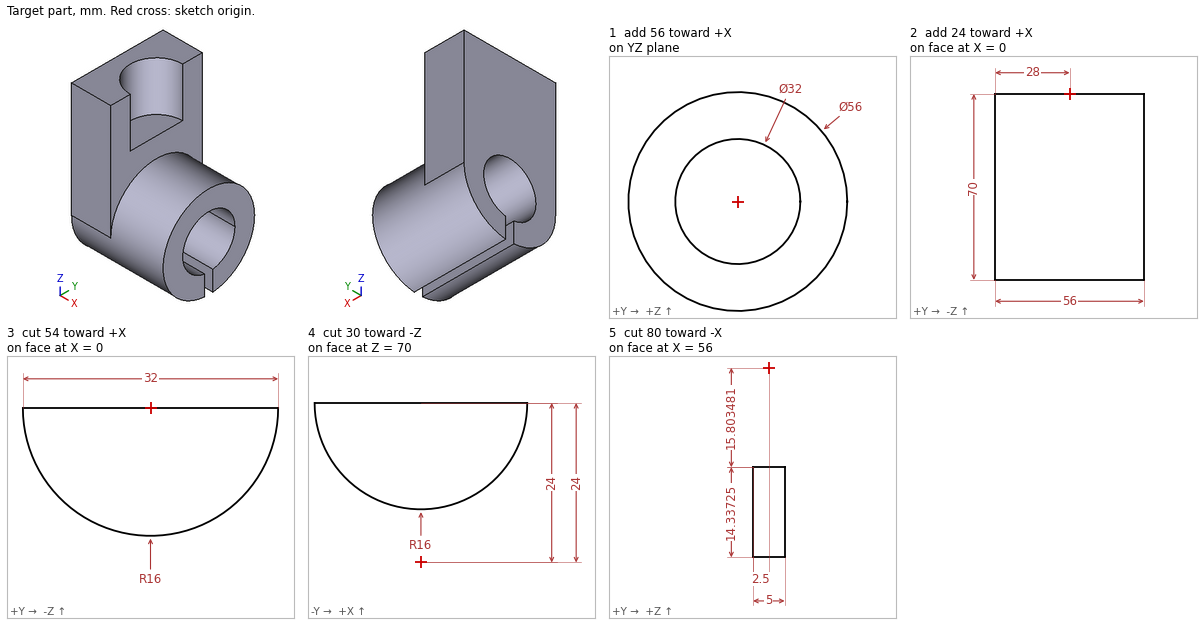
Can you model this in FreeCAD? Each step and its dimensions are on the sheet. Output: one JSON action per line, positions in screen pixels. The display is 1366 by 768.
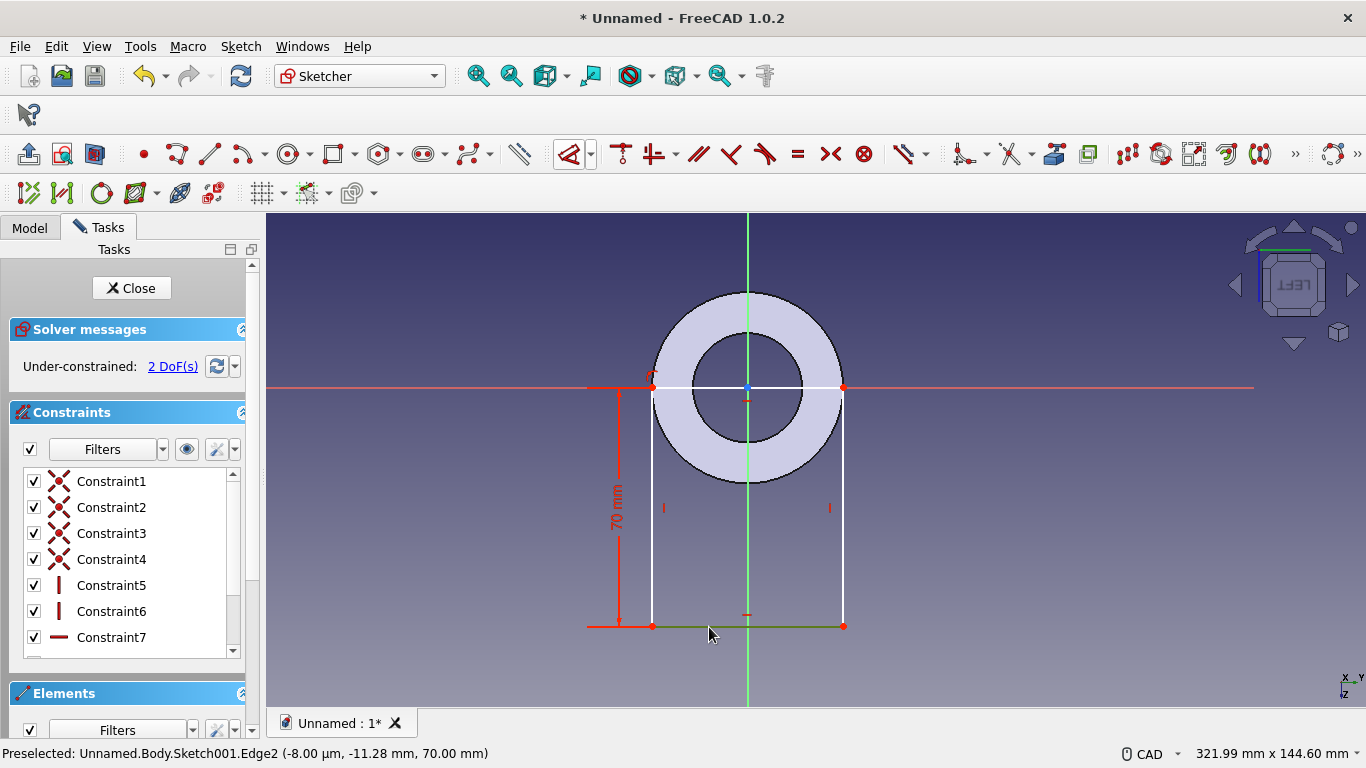
{"action": "left_click", "coordinate": [590, 154]}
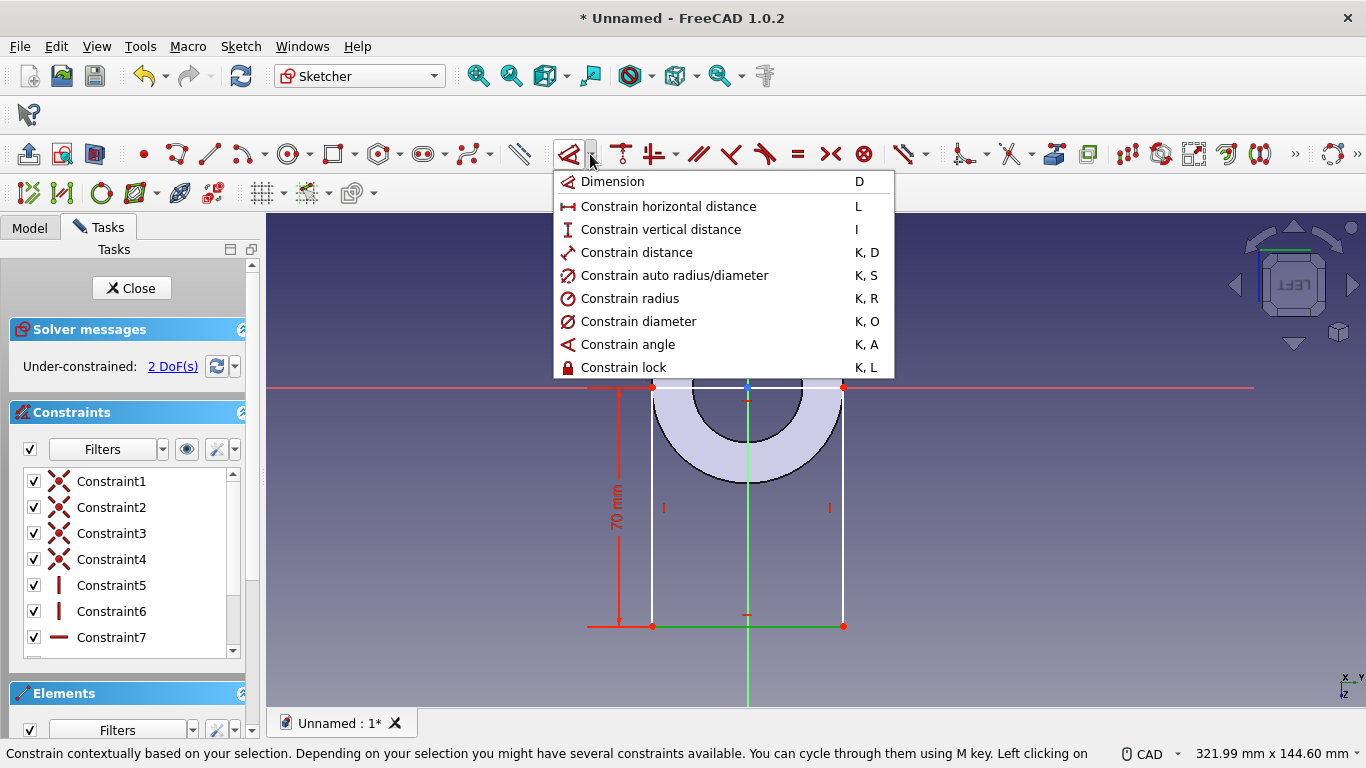
{"action": "left_click", "coordinate": [724, 206]}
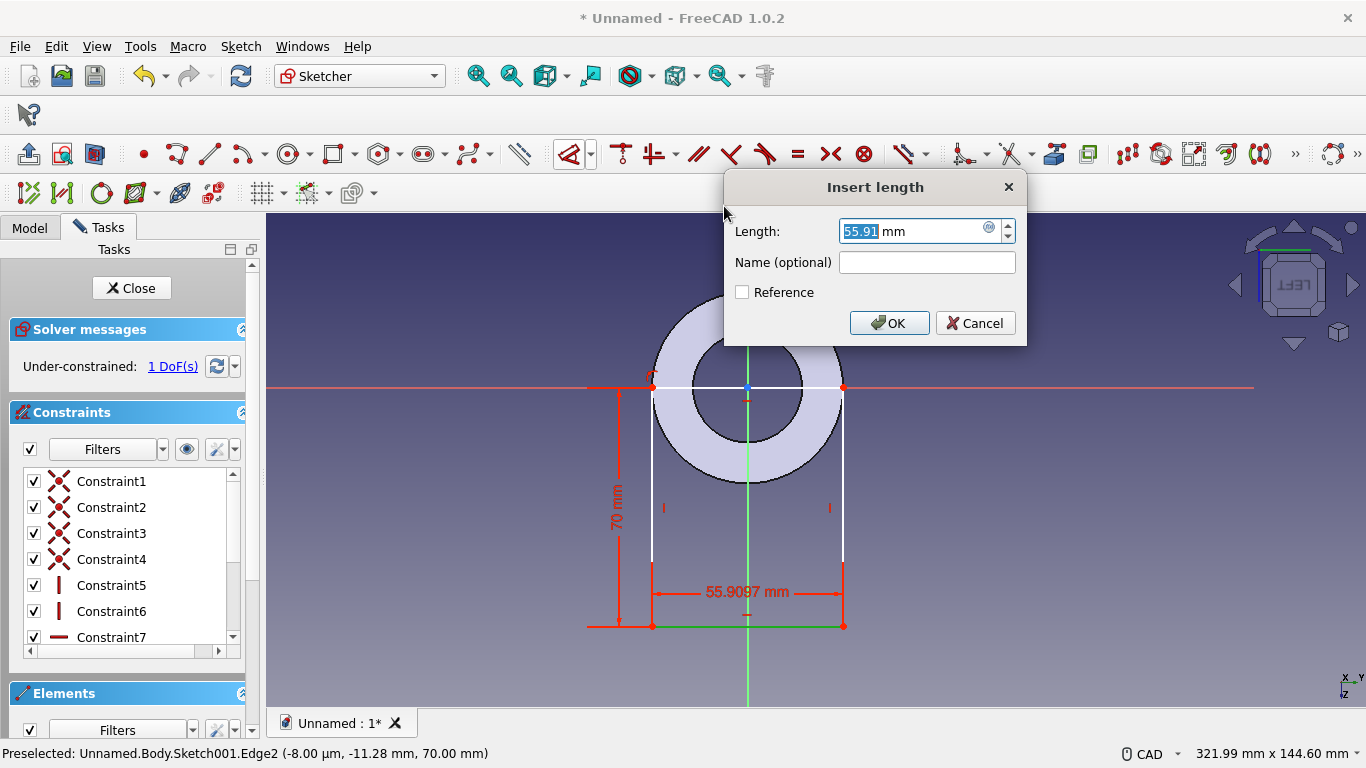
{"action": "type", "text": "56"}
{"action": "key", "text": "Return"}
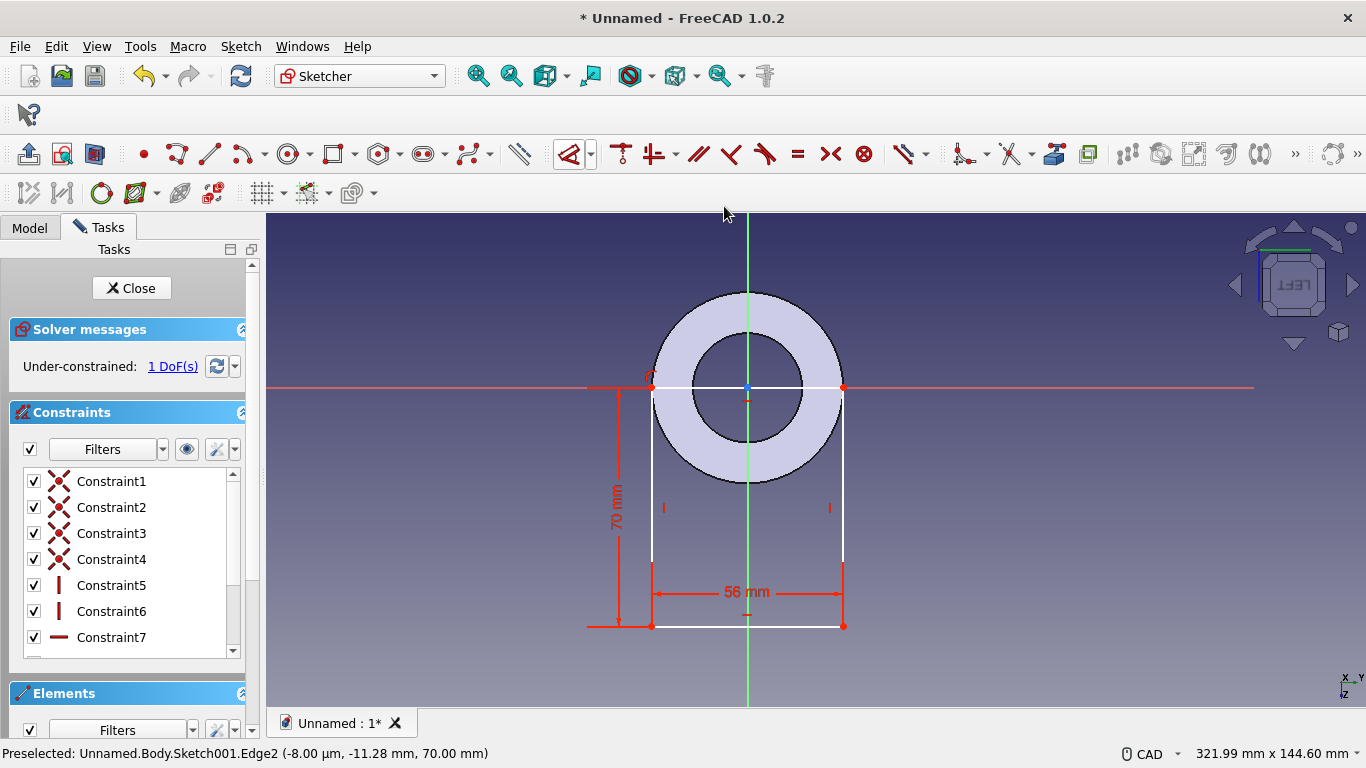
{"action": "left_click", "coordinate": [652, 388]}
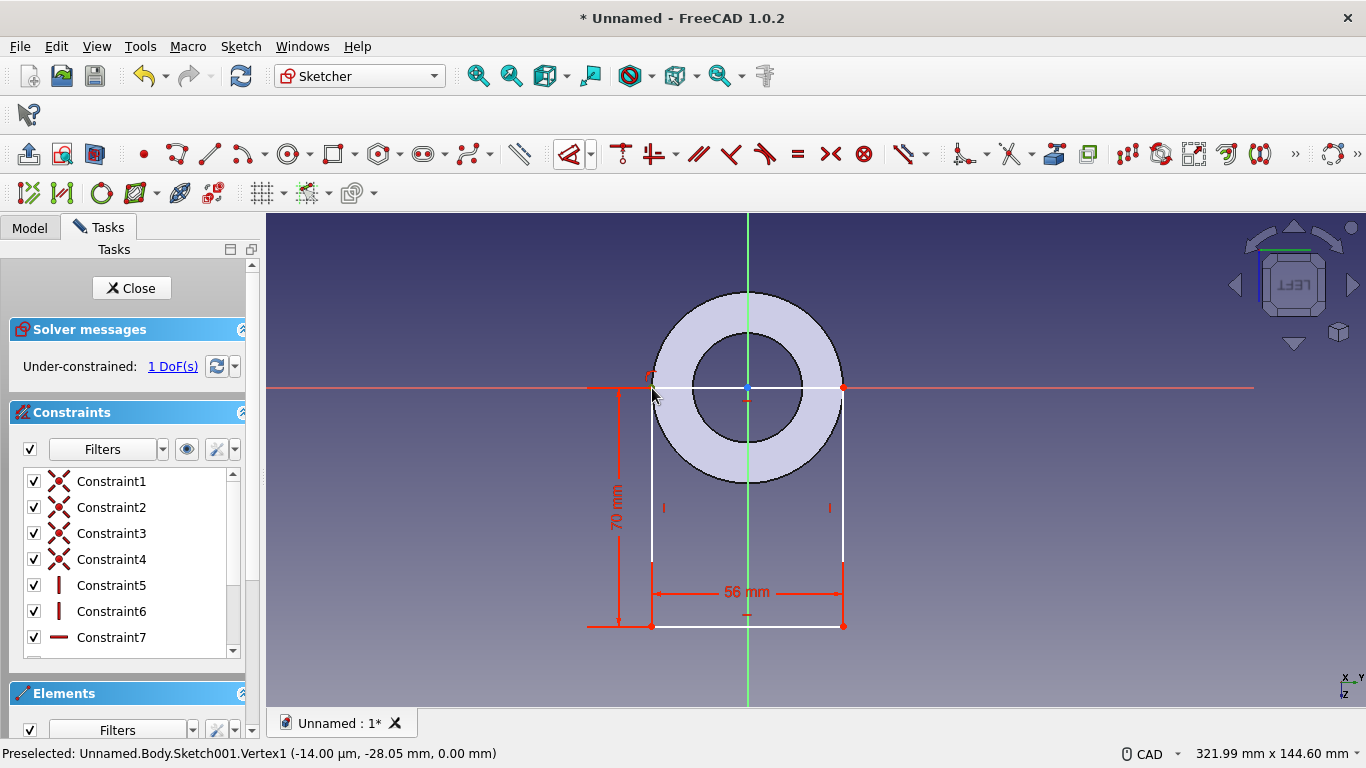
{"action": "key", "text": "l"}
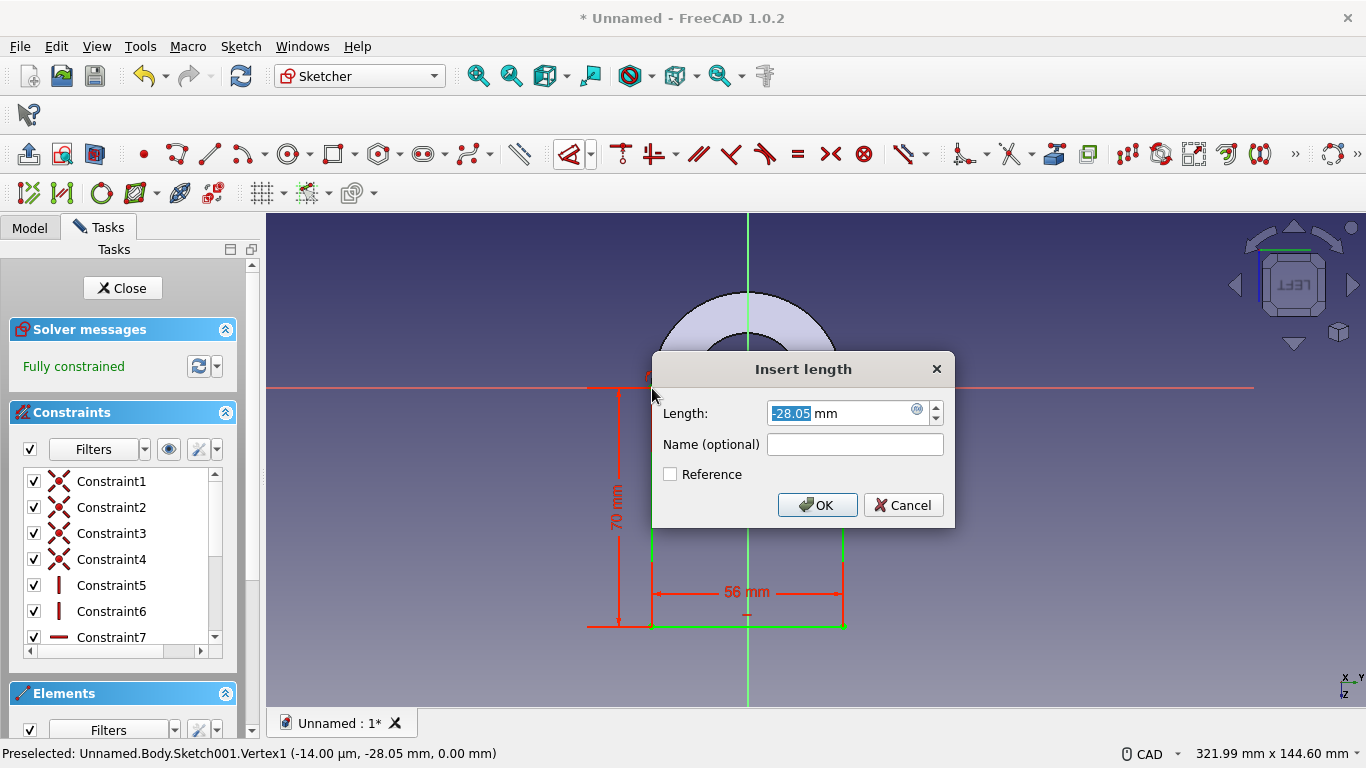
{"action": "type", "text": "-28"}
{"action": "key", "text": "Return"}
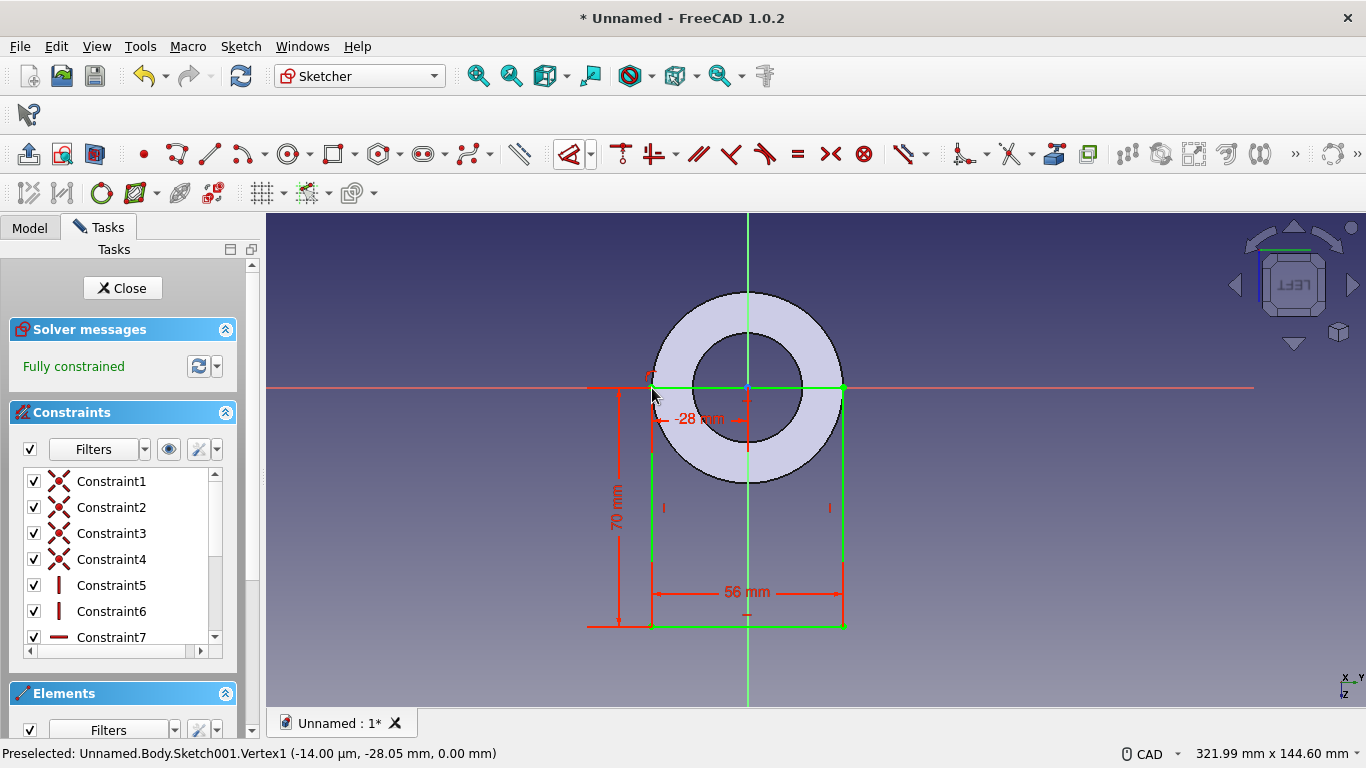
{"action": "left_click", "coordinate": [123, 288]}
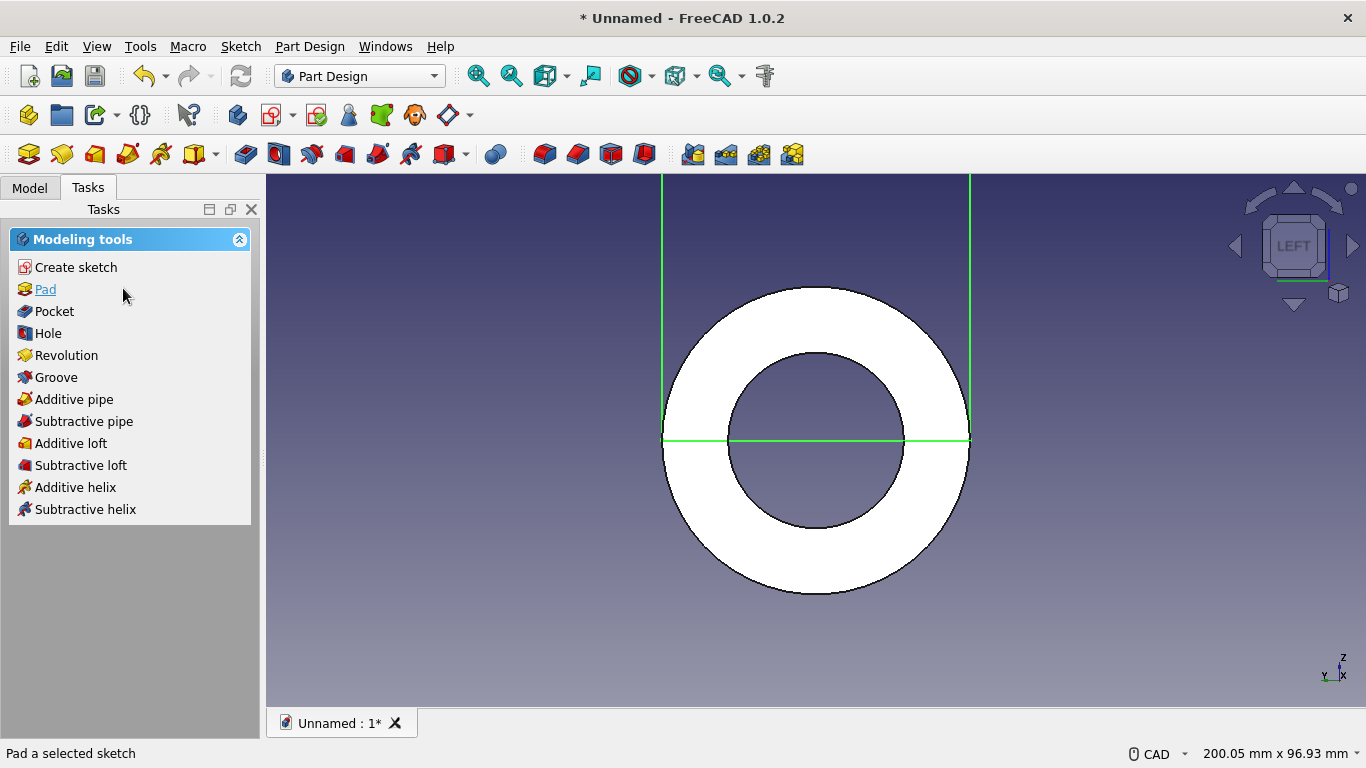
{"action": "left_click", "coordinate": [29, 154]}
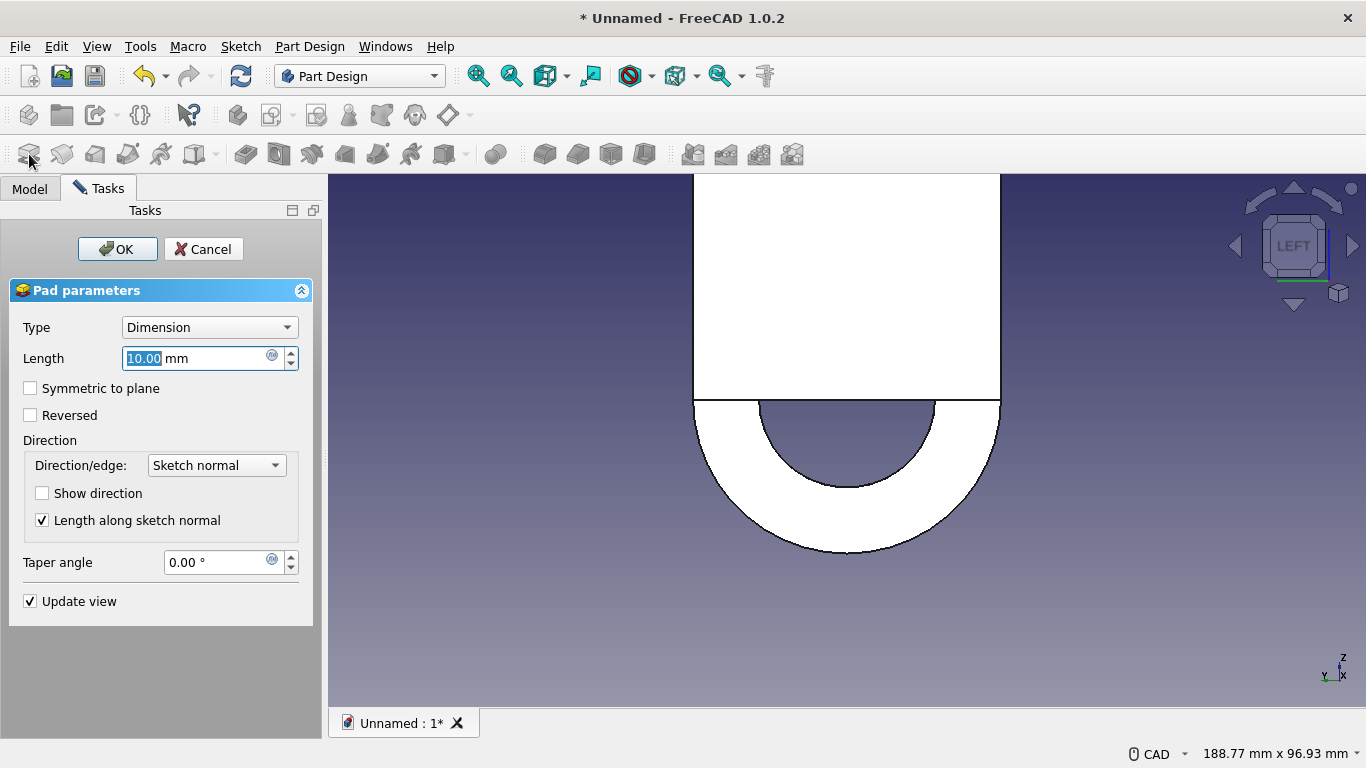
{"action": "type", "text": "24"}
{"action": "key", "text": "Tab"}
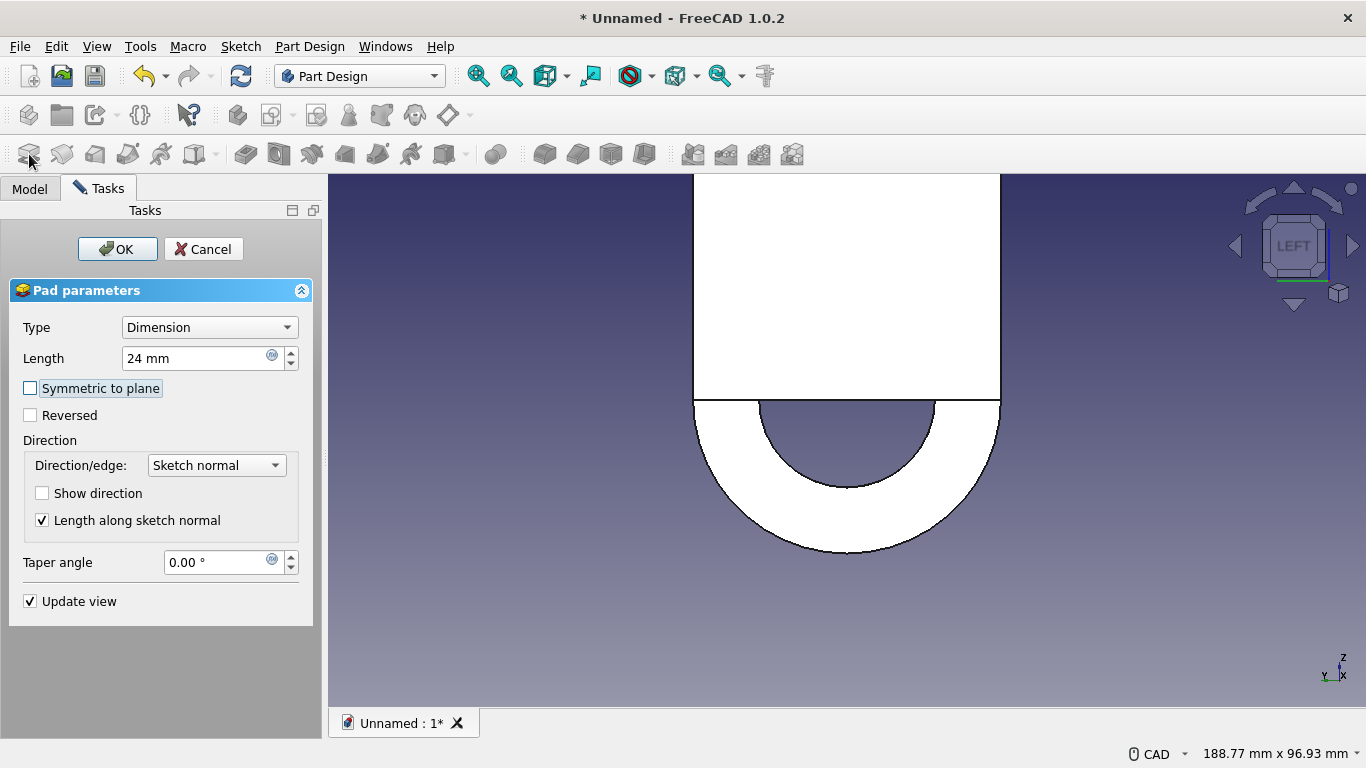
{"action": "left_click", "coordinate": [31, 415]}